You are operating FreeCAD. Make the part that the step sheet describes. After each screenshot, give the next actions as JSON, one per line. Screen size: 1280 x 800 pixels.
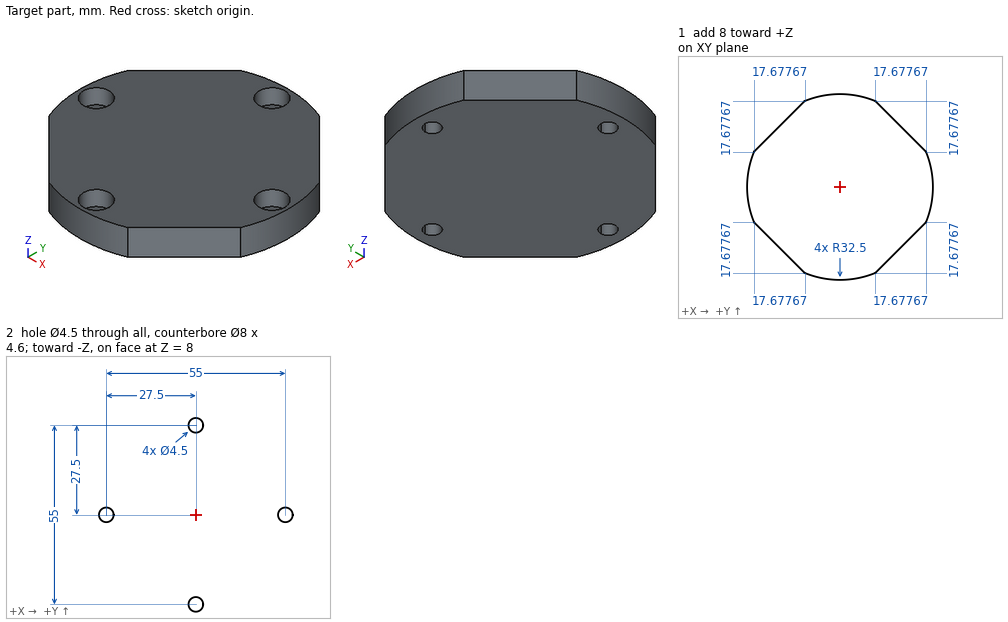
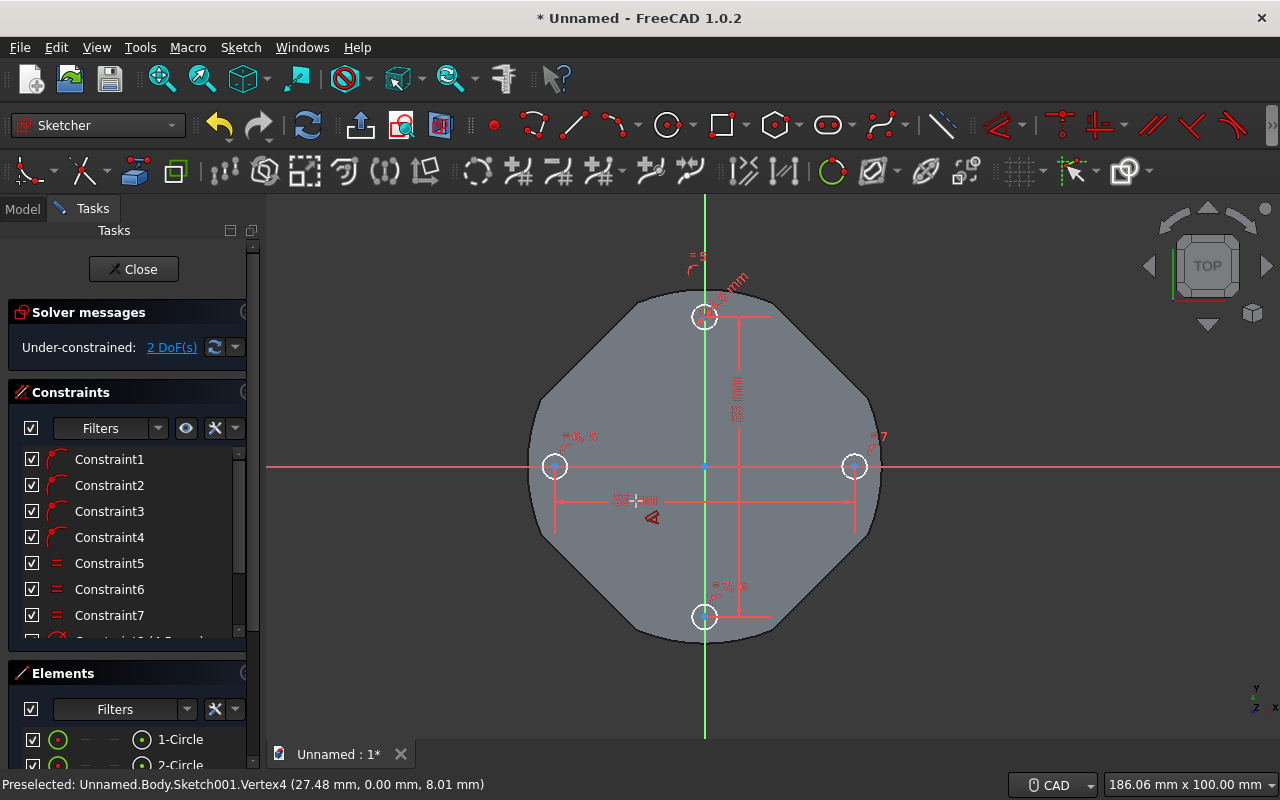
{"action": "left_click", "coordinate": [705, 317]}
{"action": "left_click", "coordinate": [739, 358]}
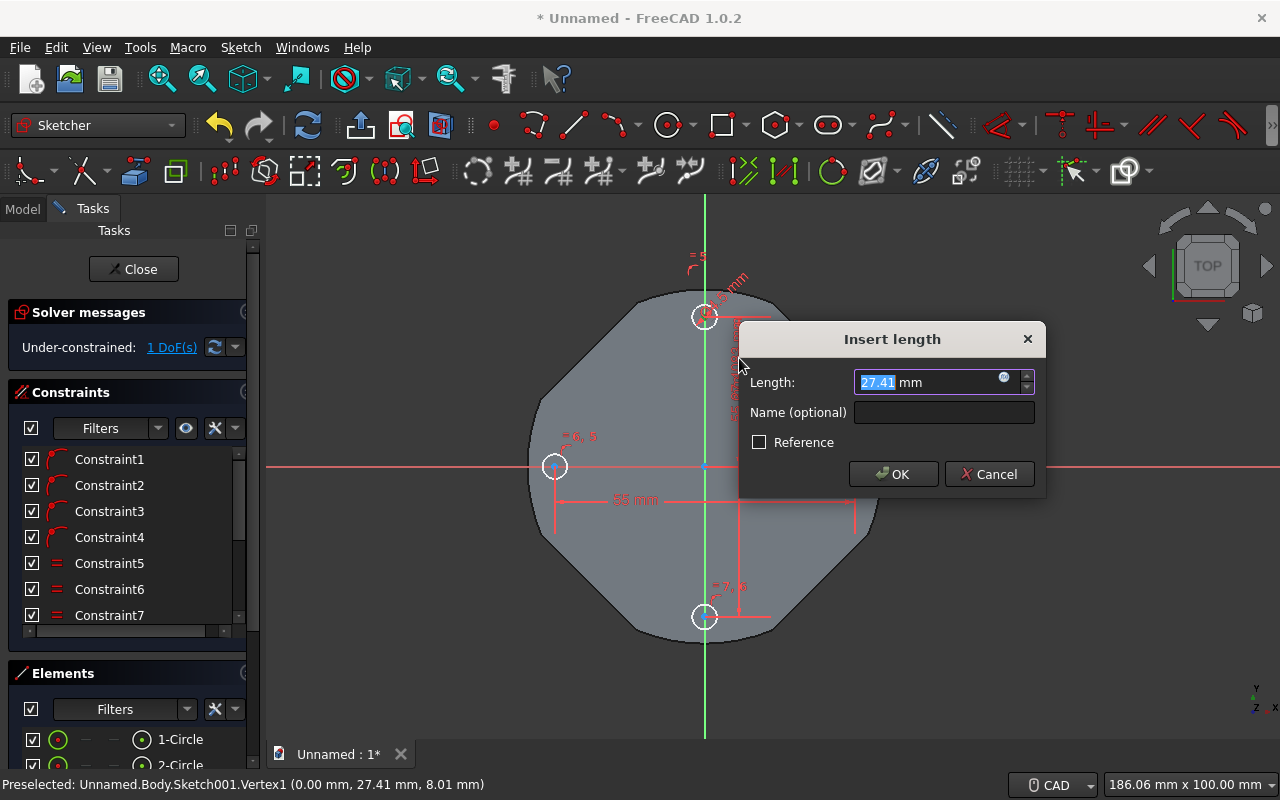
{"action": "type", "text": "27.5"}
{"action": "key", "text": "Return"}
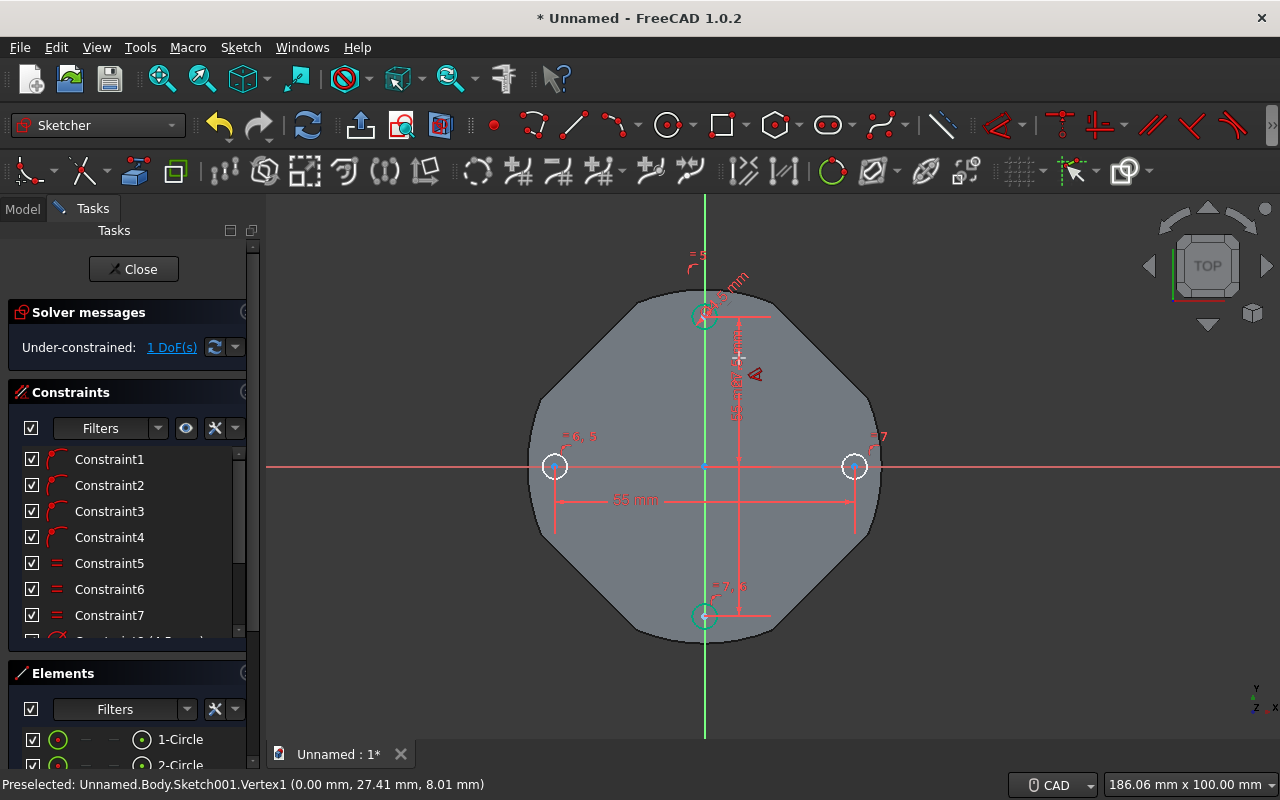
{"action": "left_click", "coordinate": [555, 467]}
{"action": "left_click", "coordinate": [630, 433]}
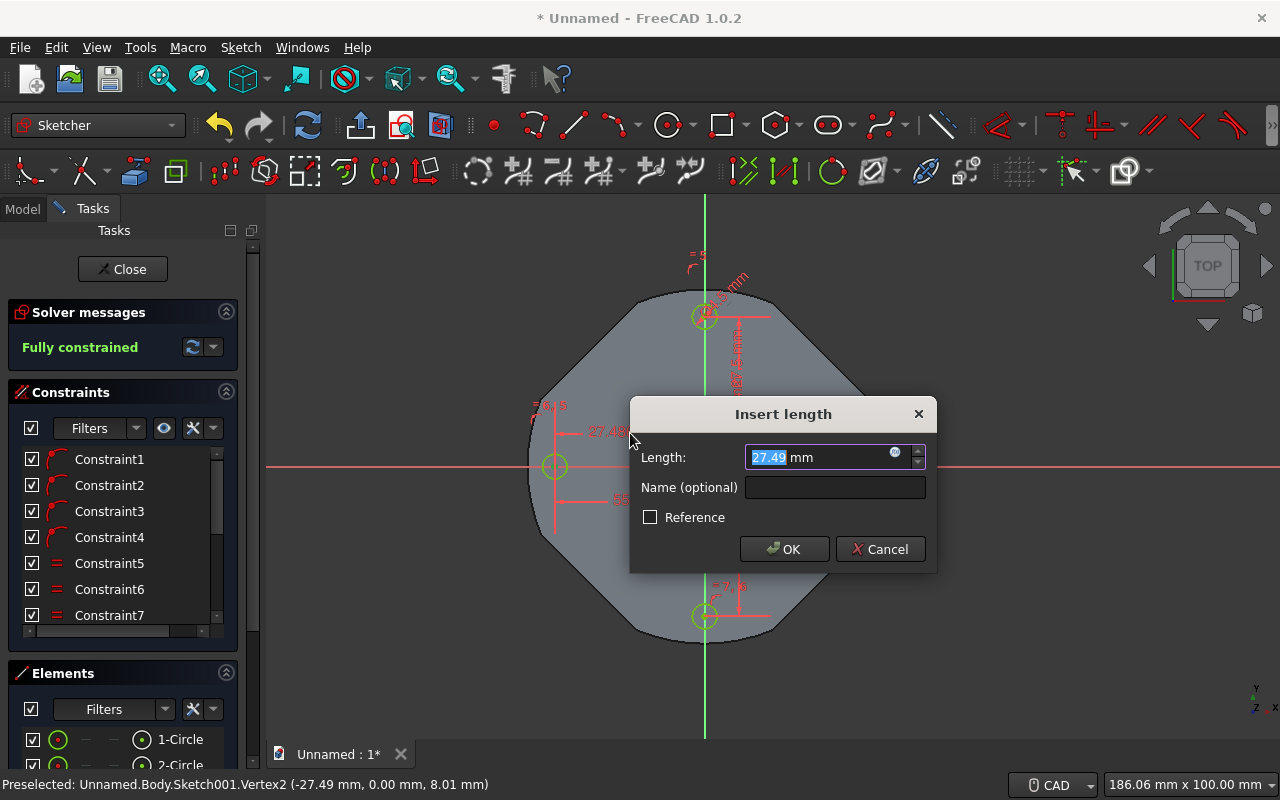
{"action": "type", "text": "27.5"}
{"action": "key", "text": "Return"}
{"action": "key", "text": "Escape"}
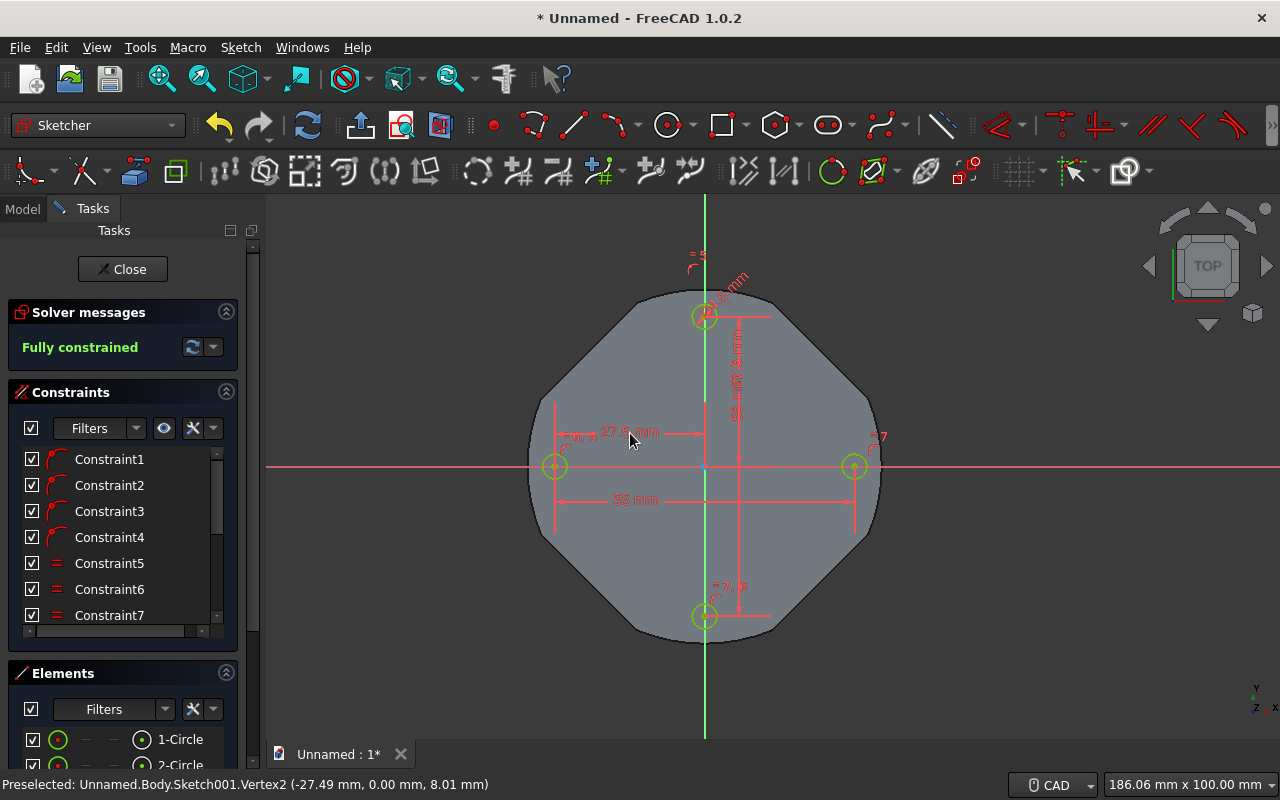
{"action": "left_click", "coordinate": [123, 269]}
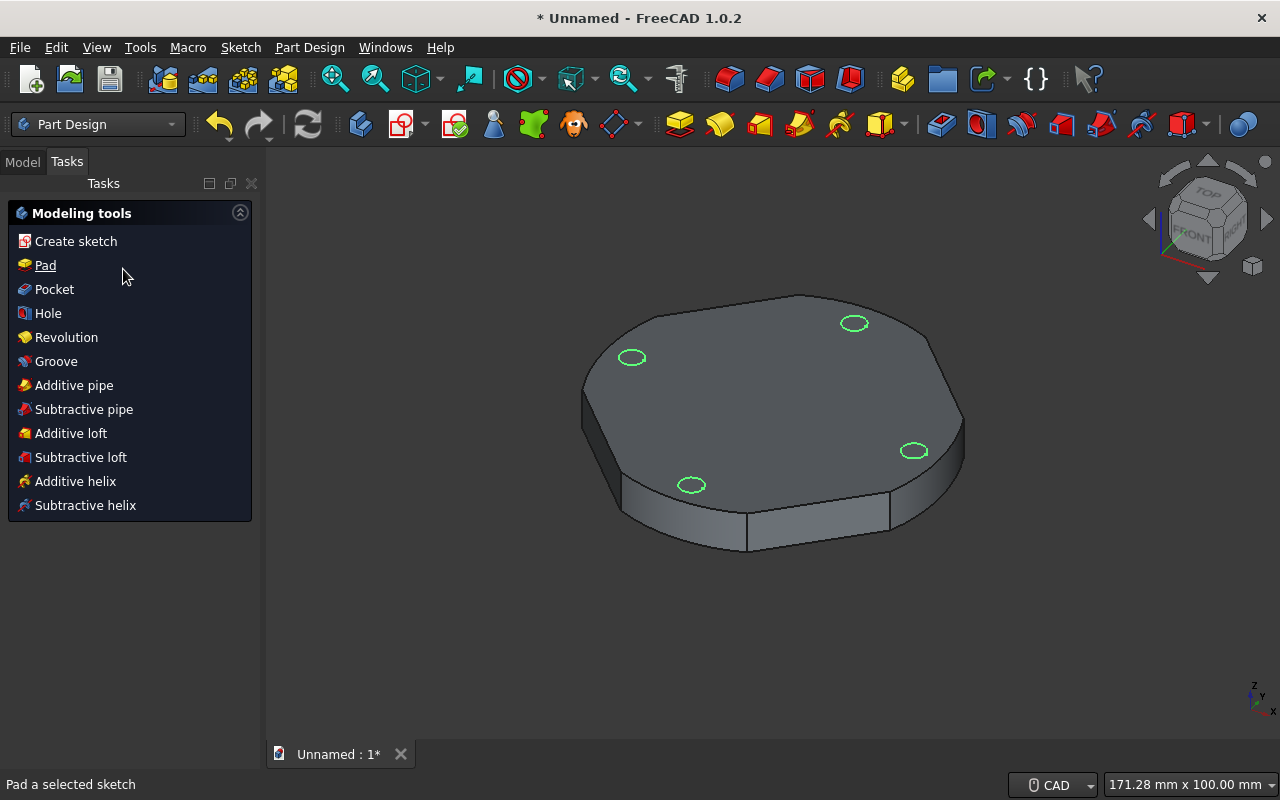
{"action": "left_click", "coordinate": [982, 124]}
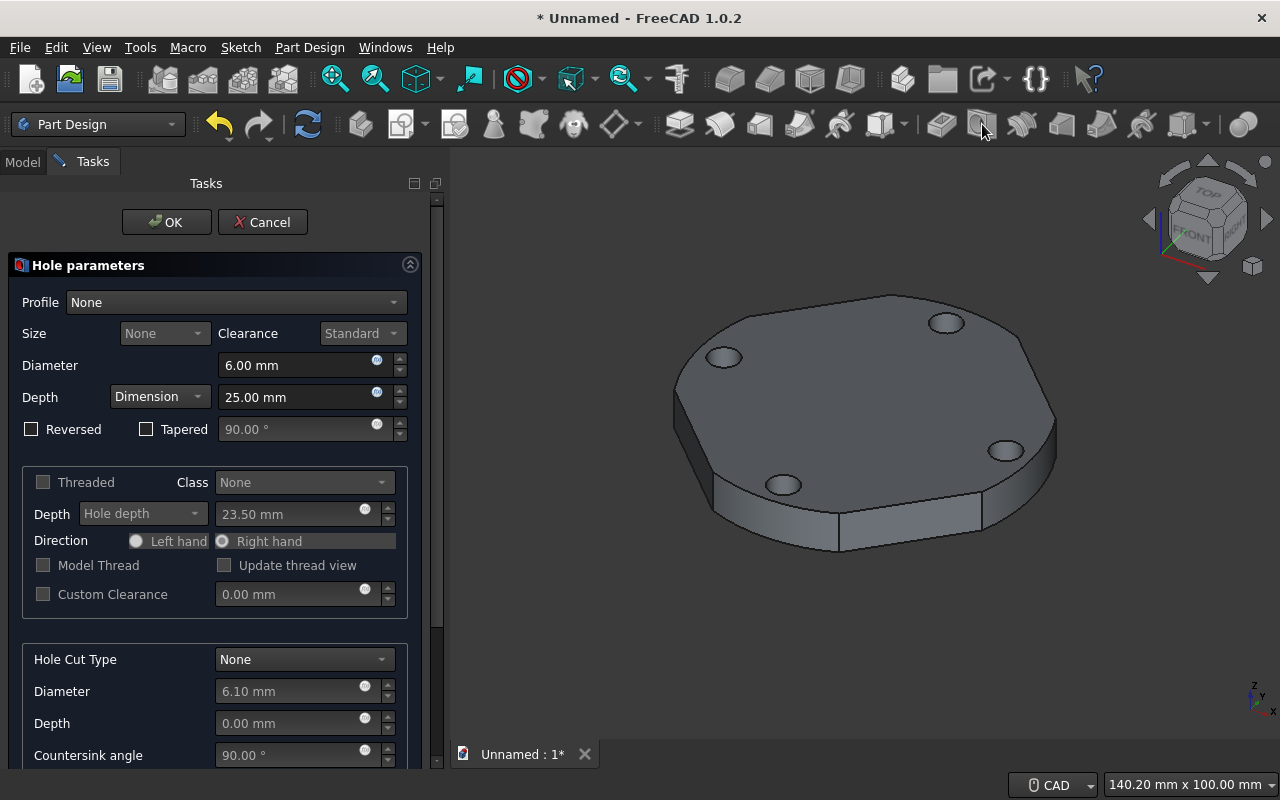
{"action": "triple_click", "coordinate": [305, 365]}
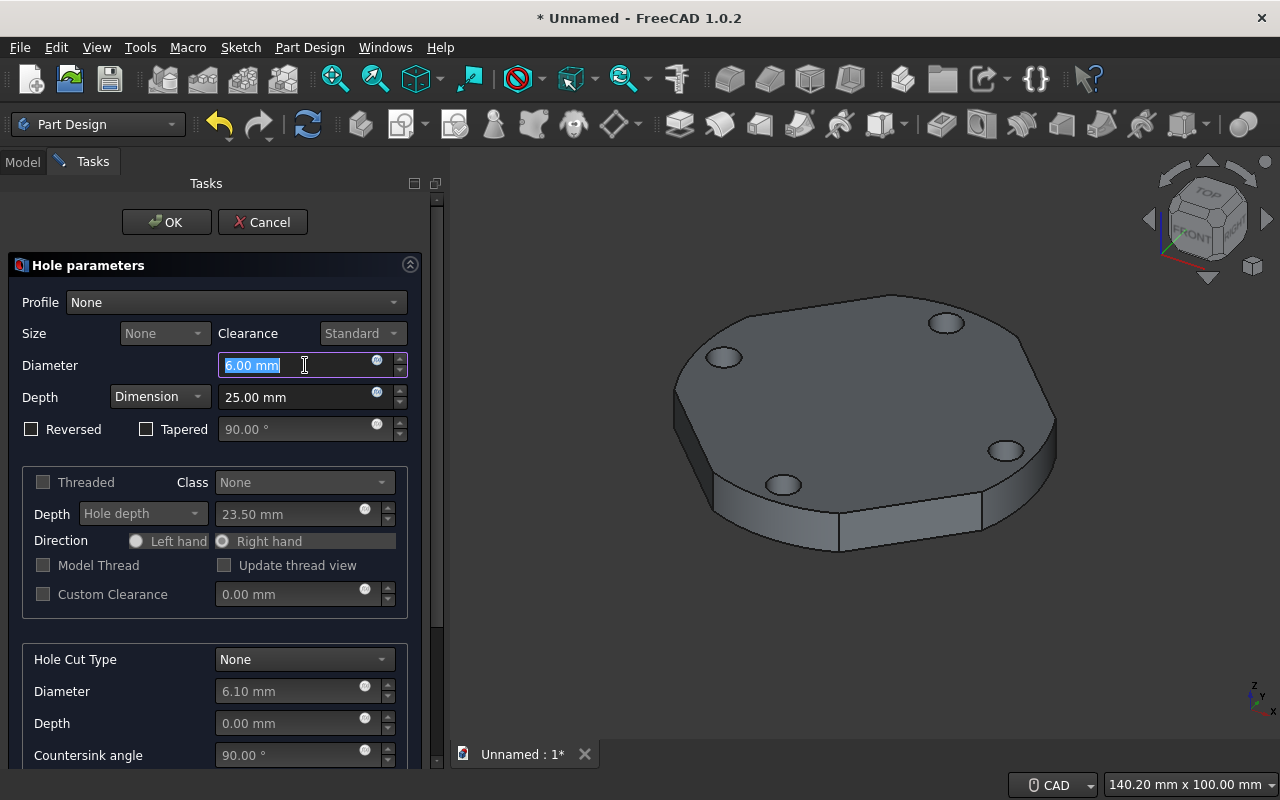
{"action": "type", "text": "4.5"}
{"action": "key", "text": "Tab"}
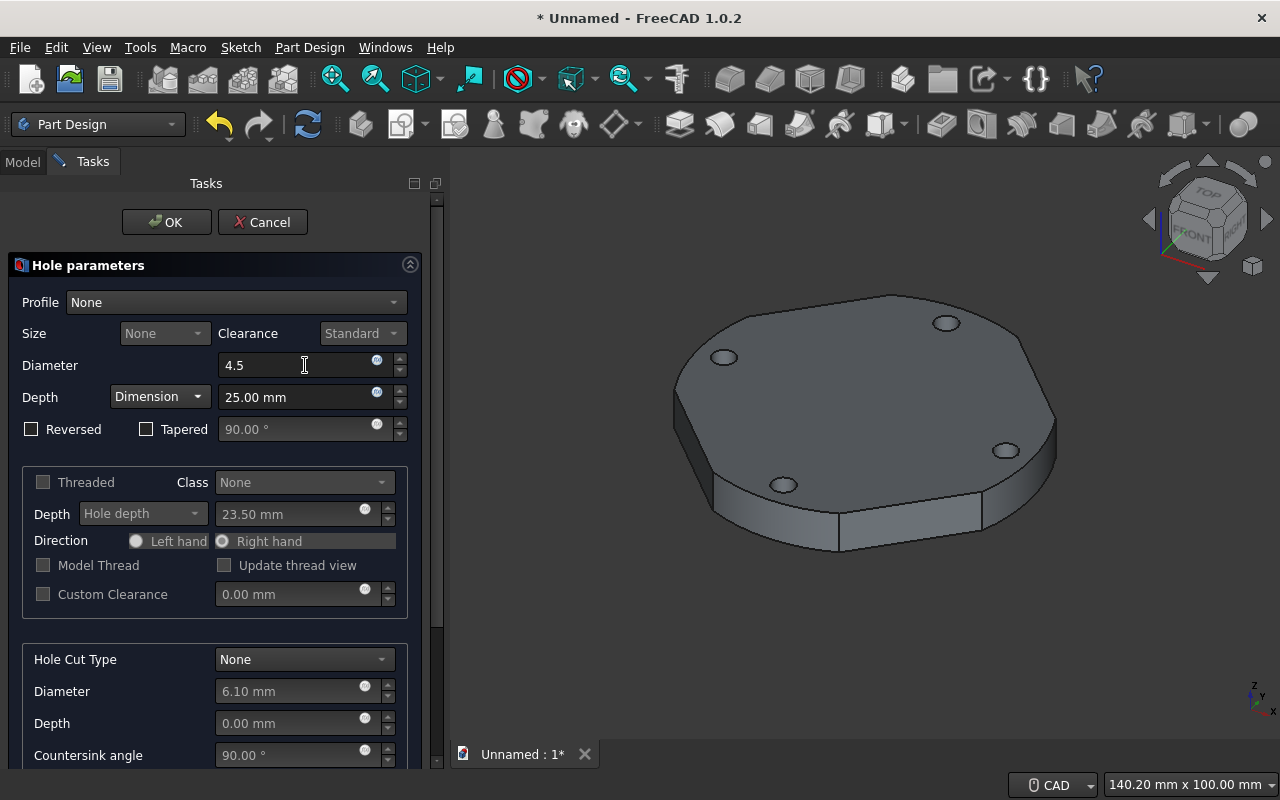
{"action": "left_click", "coordinate": [161, 396]}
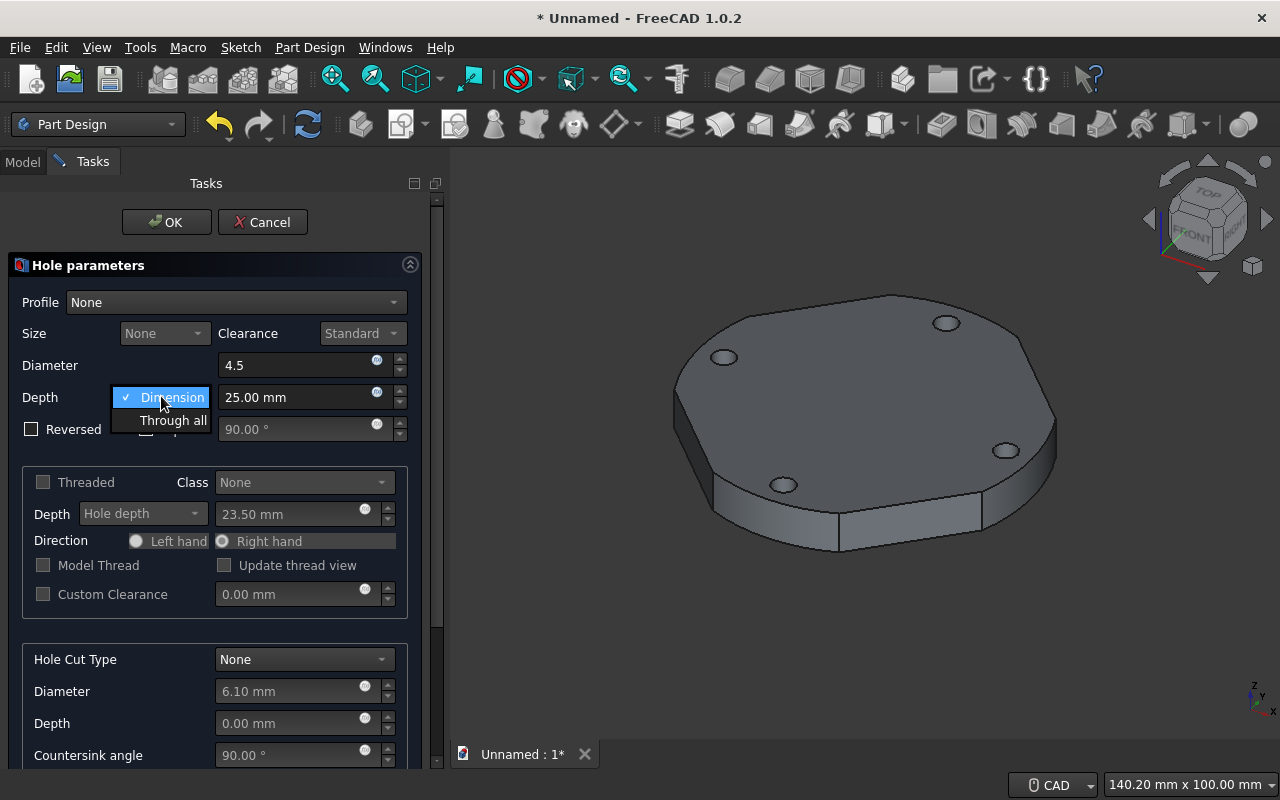
{"action": "left_click", "coordinate": [160, 420]}